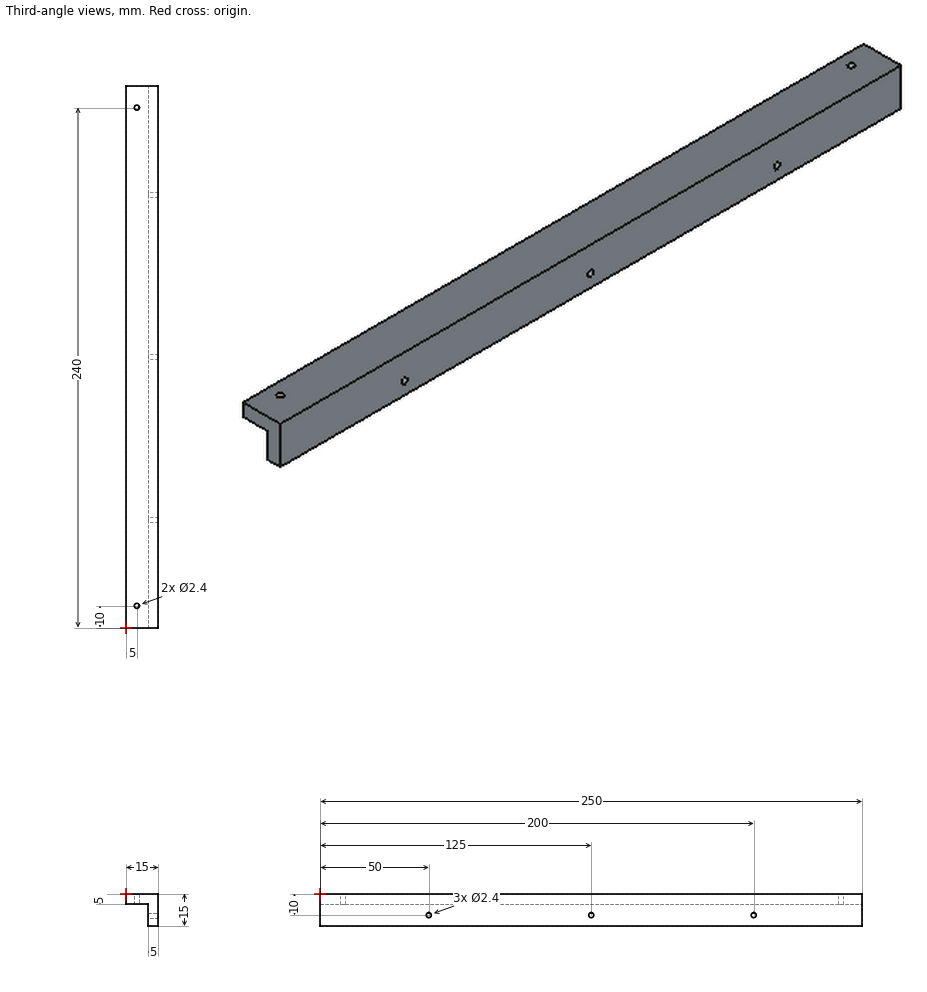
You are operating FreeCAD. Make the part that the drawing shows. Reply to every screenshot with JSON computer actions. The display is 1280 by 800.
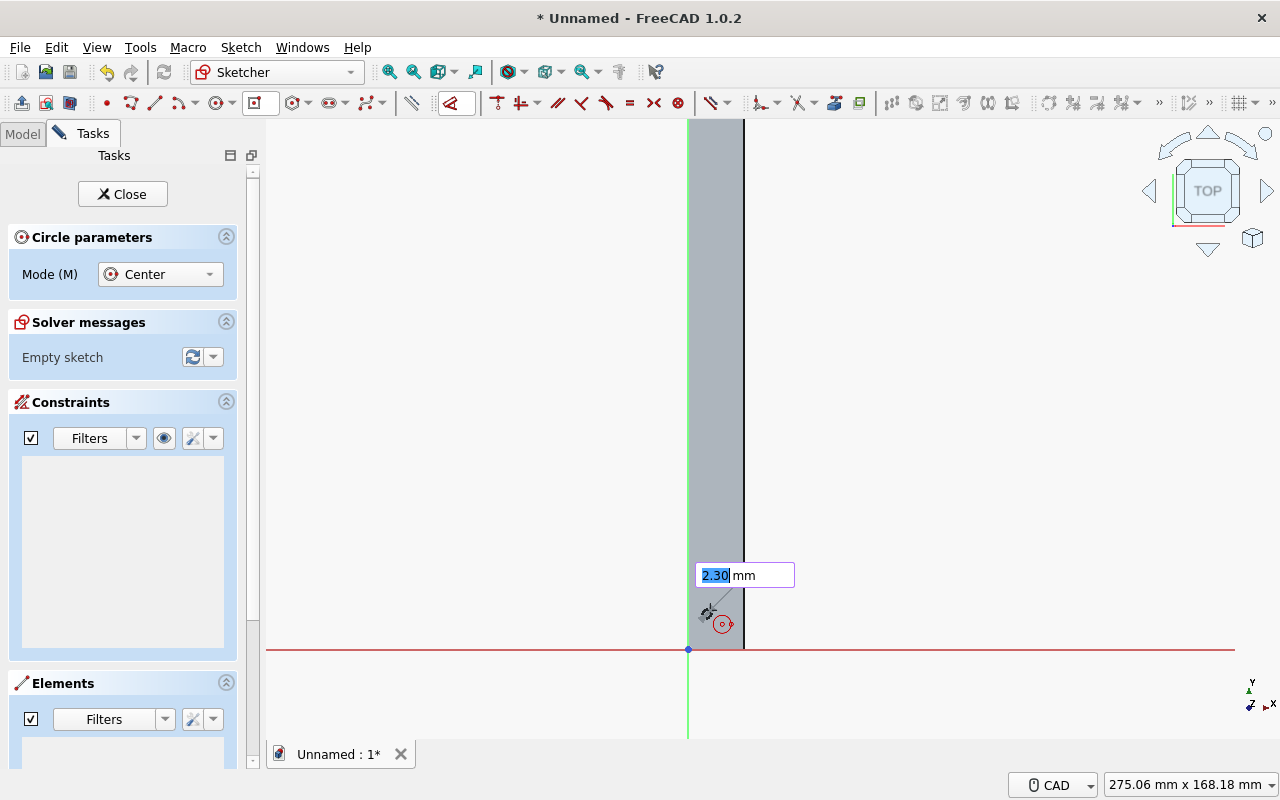
{"action": "type", "text": "2.4"}
{"action": "key", "text": "Return"}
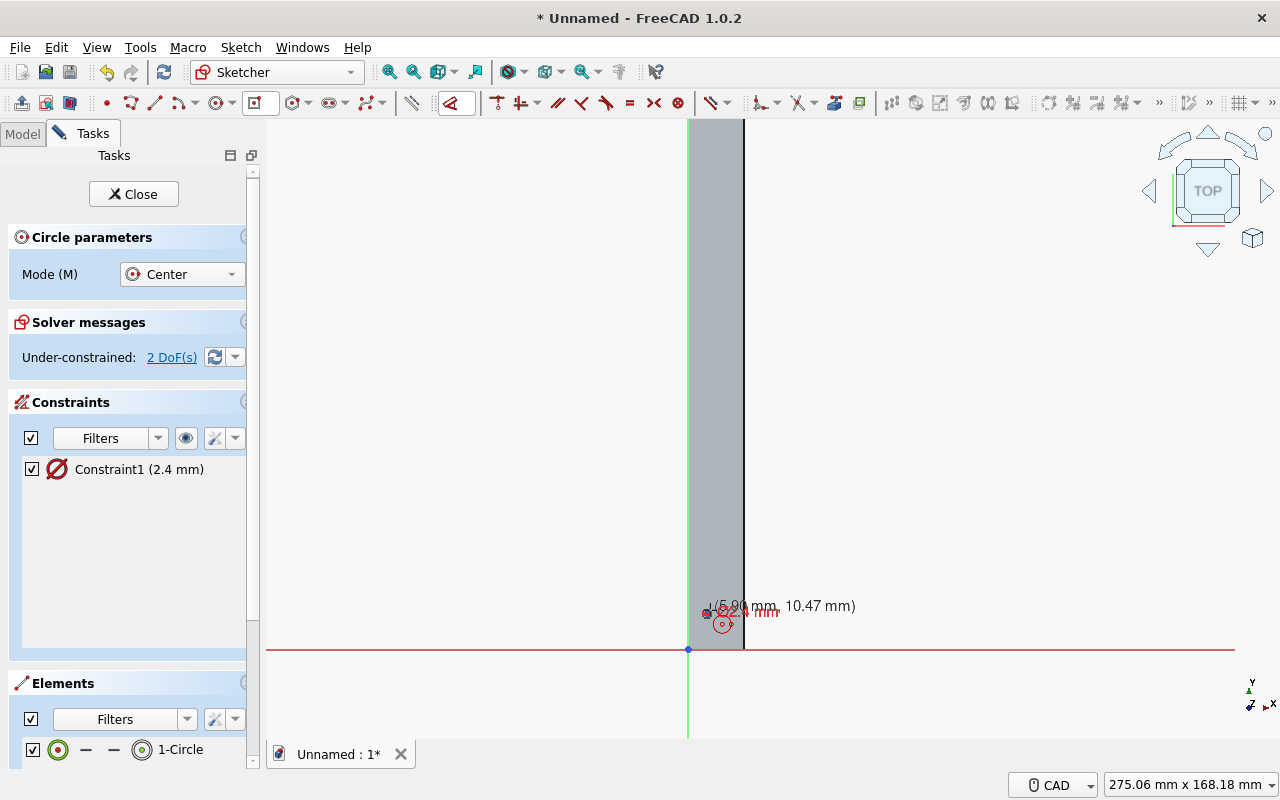
{"action": "scroll", "coordinate": [708, 612], "scroll_direction": "down", "scroll_amount": 4}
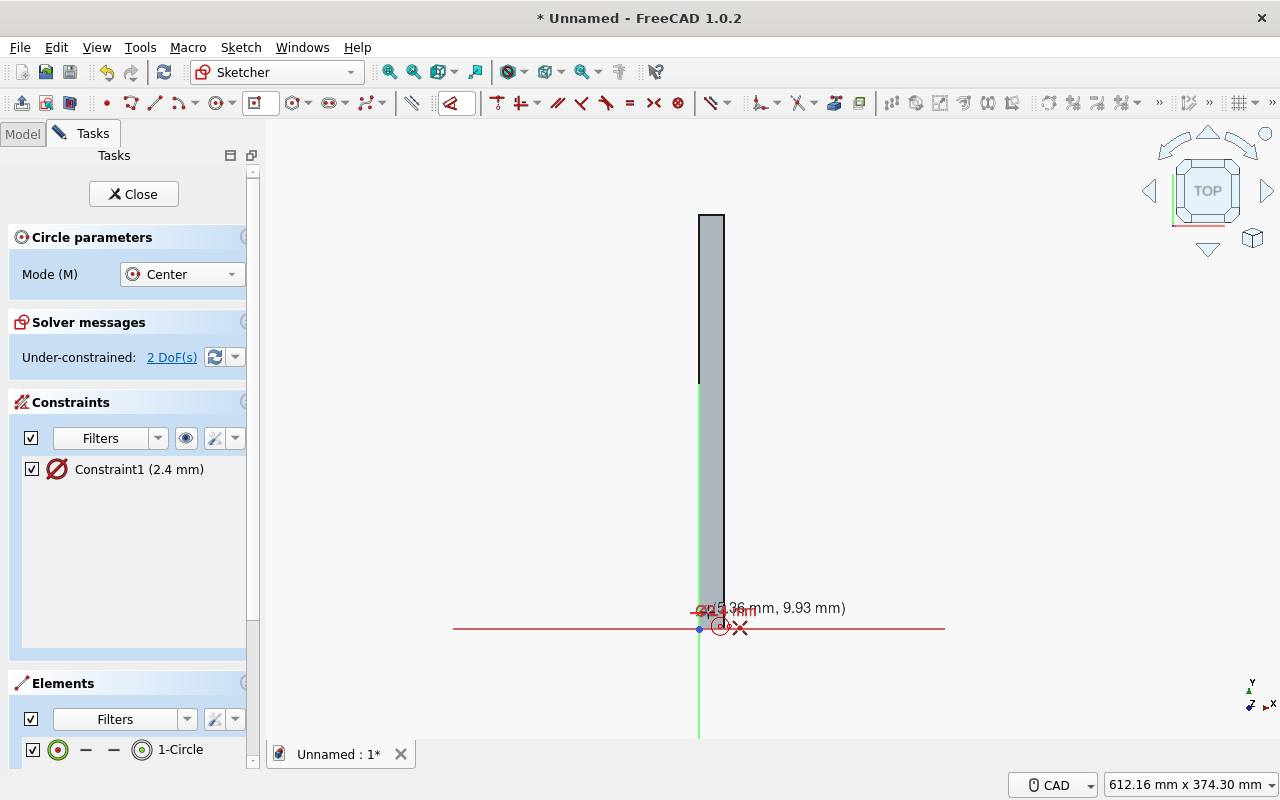
{"action": "scroll", "coordinate": [708, 232], "scroll_direction": "up", "scroll_amount": 13}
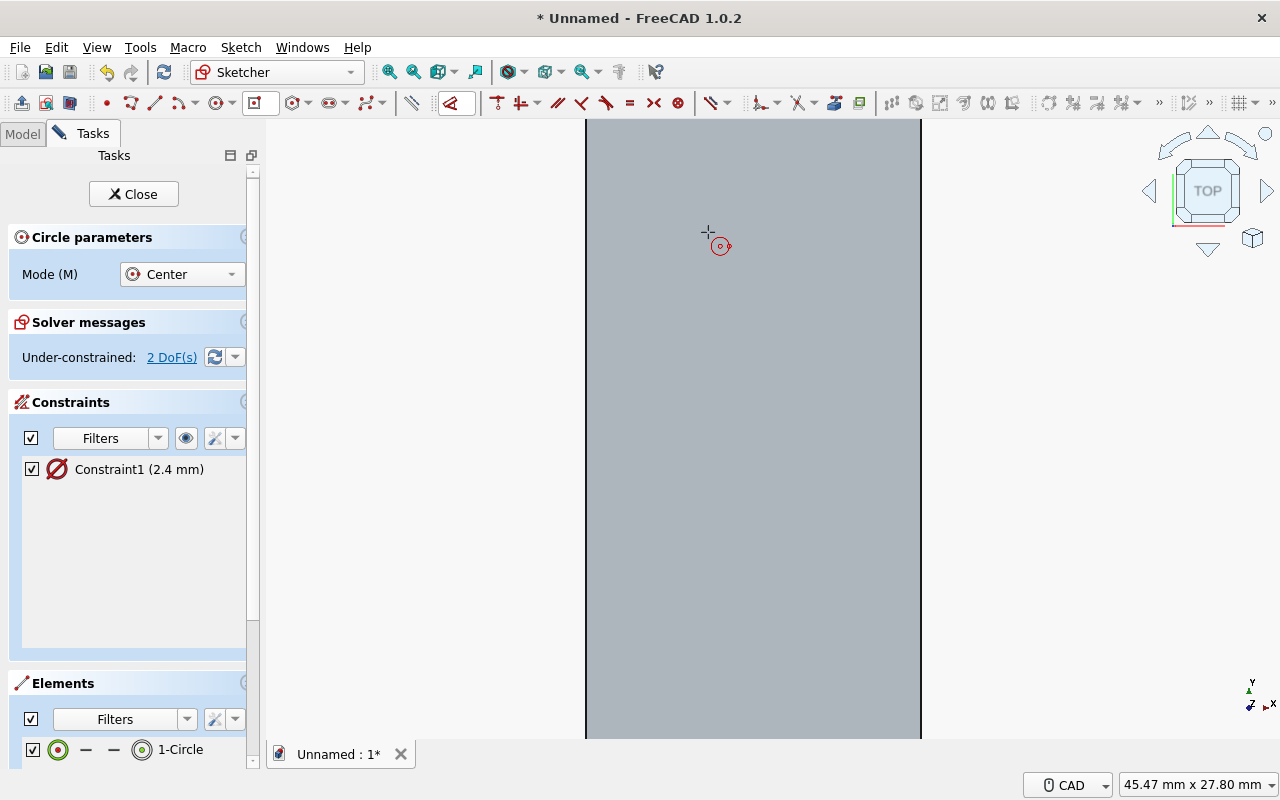
{"action": "scroll", "coordinate": [708, 232], "scroll_direction": "down", "scroll_amount": 13}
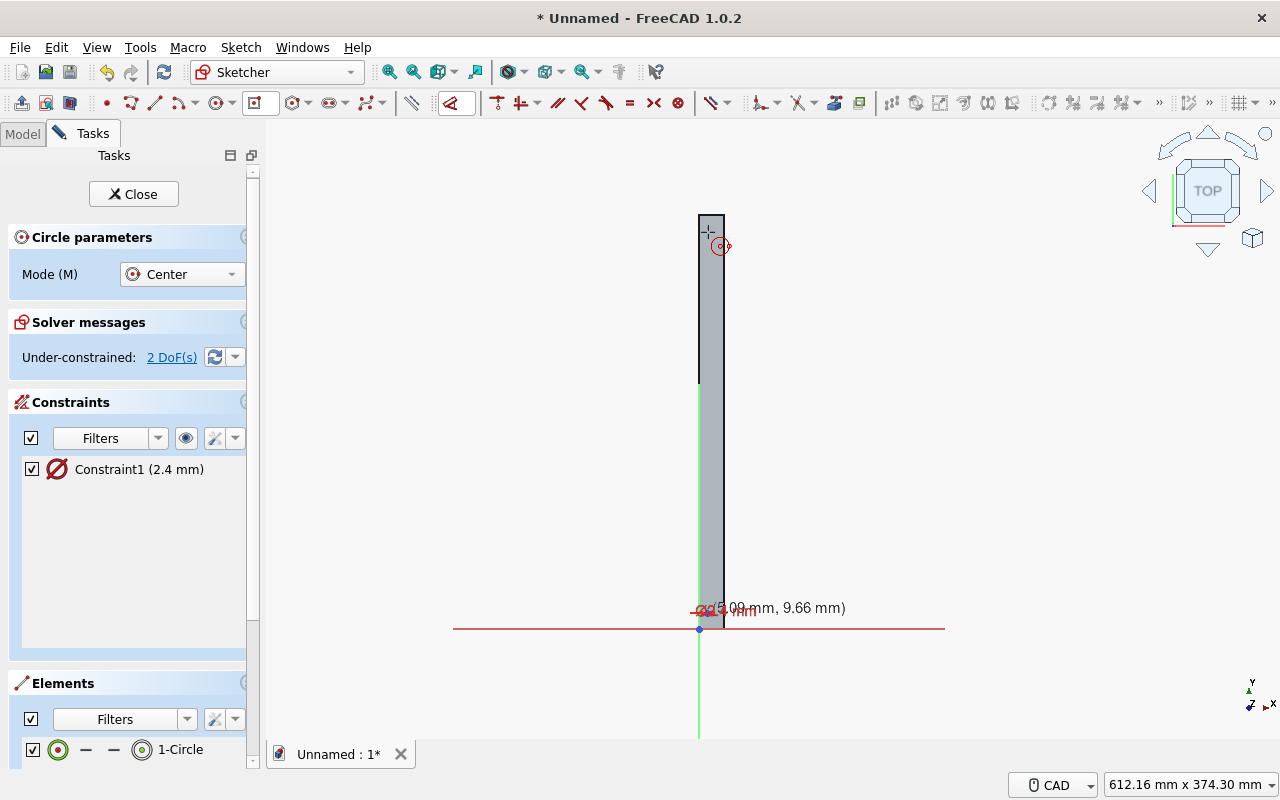
{"action": "scroll", "coordinate": [708, 232], "scroll_direction": "up", "scroll_amount": 4}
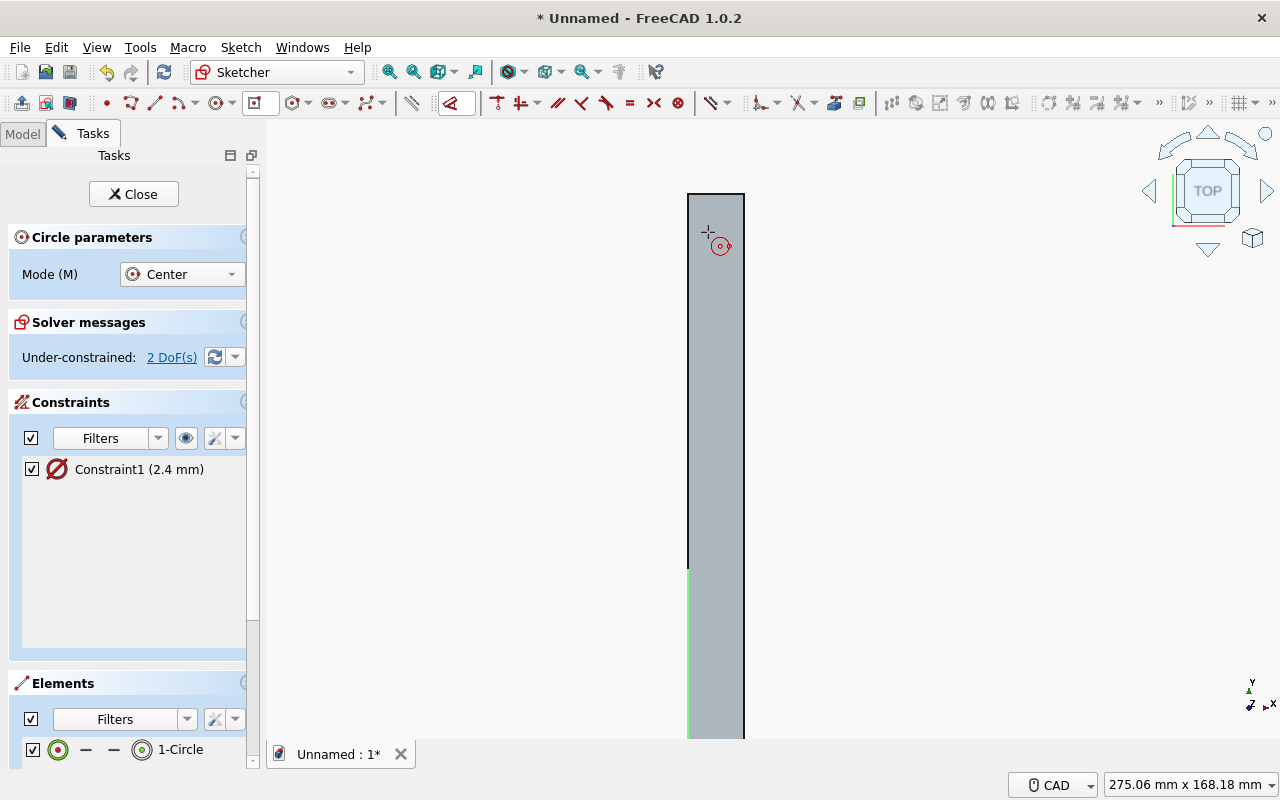
{"action": "left_click", "coordinate": [707, 231]}
{"action": "mouse_move", "coordinate": [710, 228]}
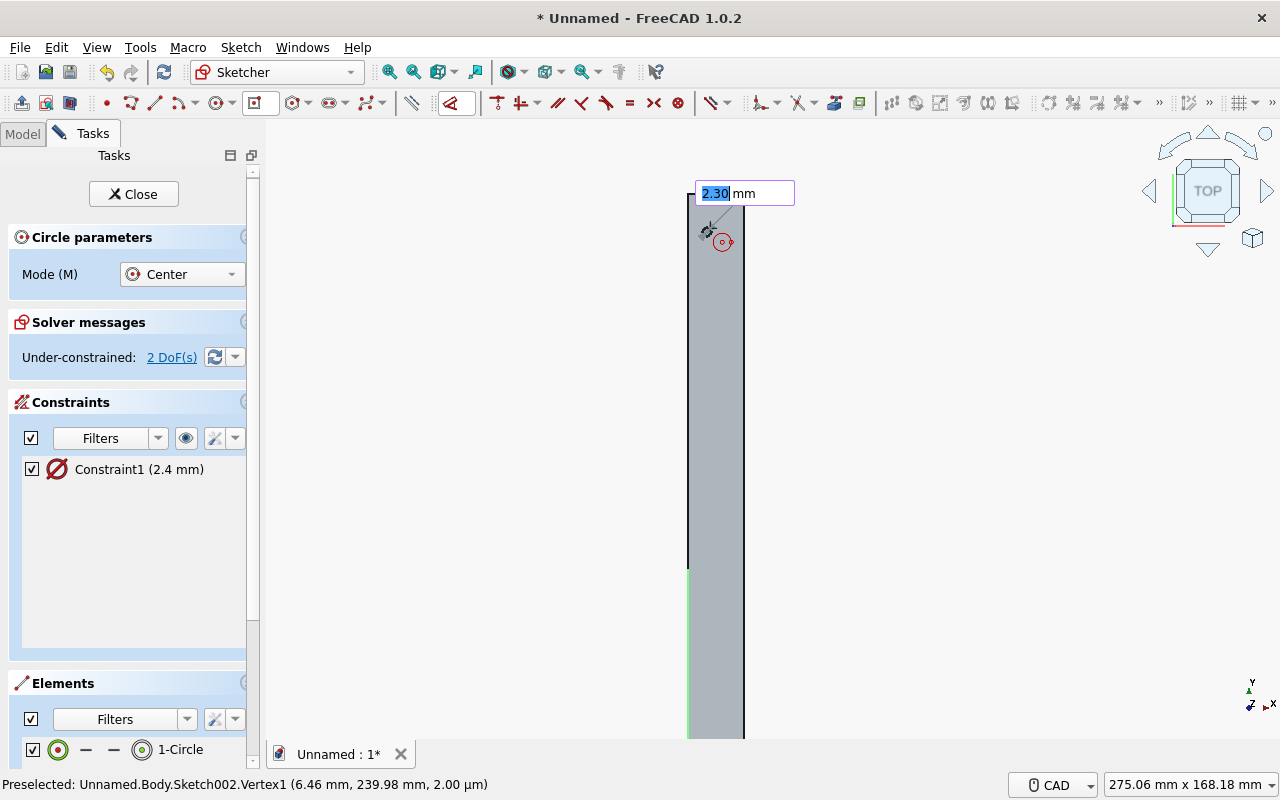
{"action": "type", "text": "2.4"}
{"action": "key", "text": "Return"}
{"action": "key", "text": "Escape"}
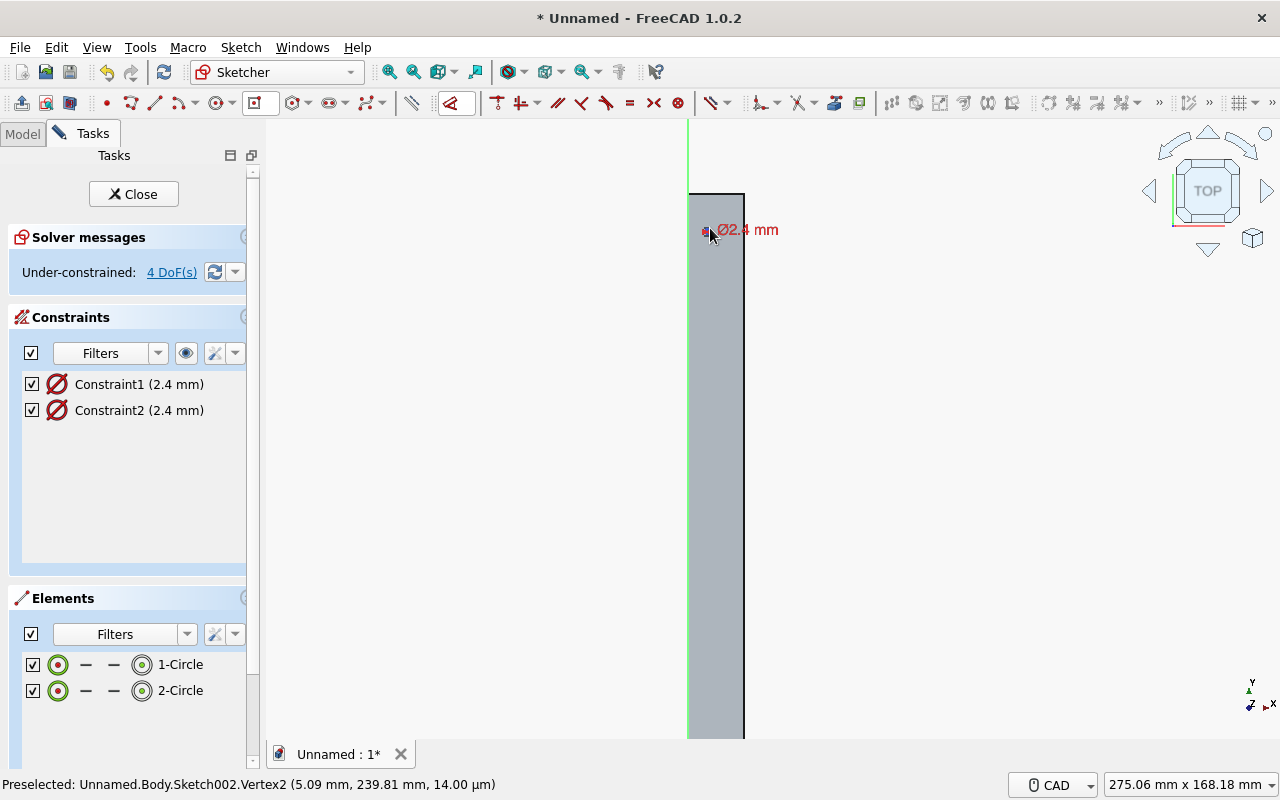
{"action": "key", "text": "d"}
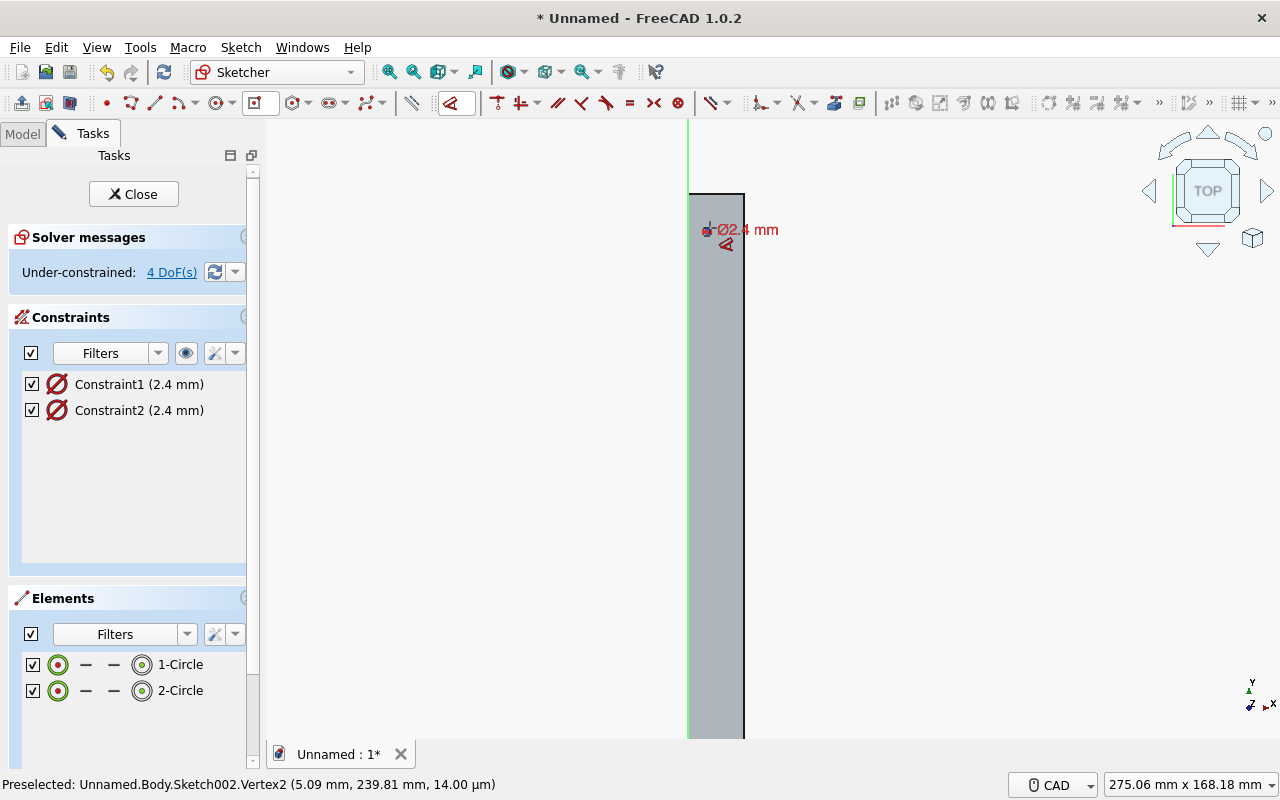
{"action": "scroll", "coordinate": [708, 231], "scroll_direction": "down", "scroll_amount": 4}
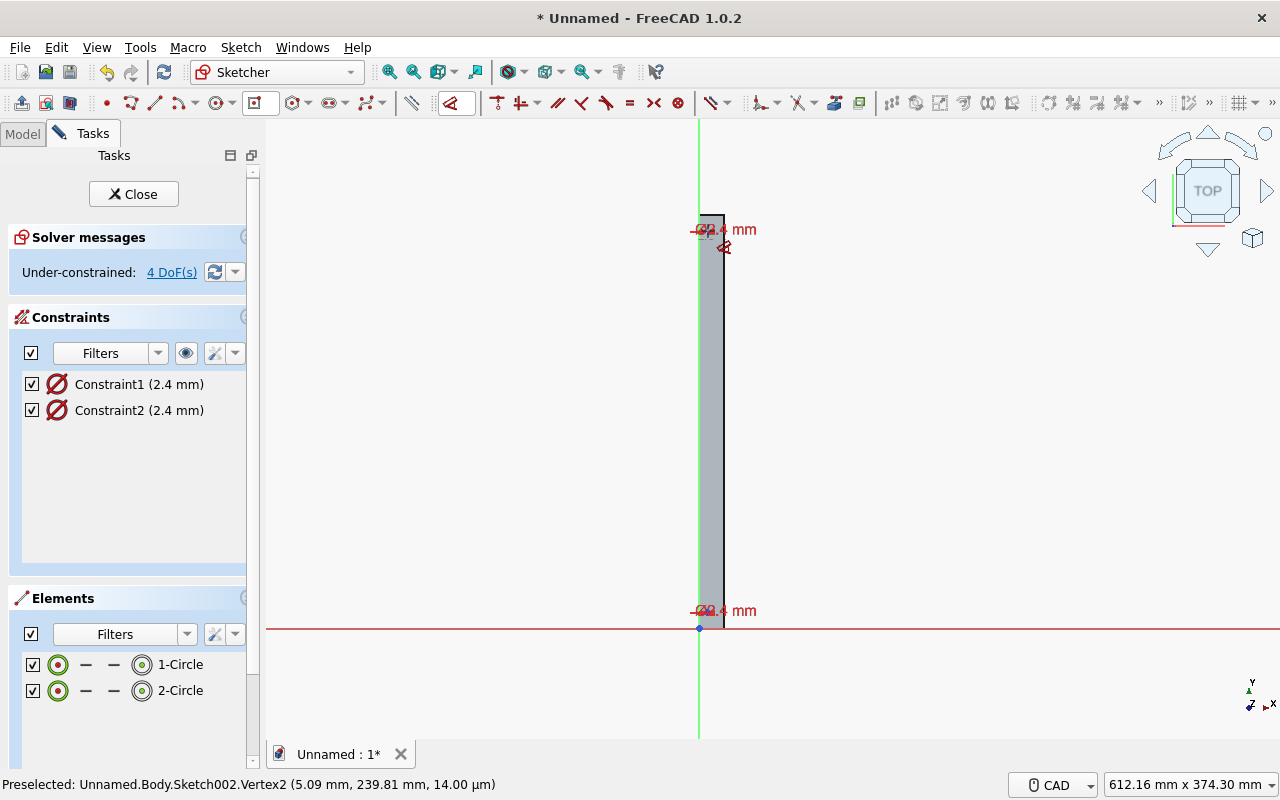
{"action": "scroll", "coordinate": [708, 613], "scroll_direction": "up", "scroll_amount": 8}